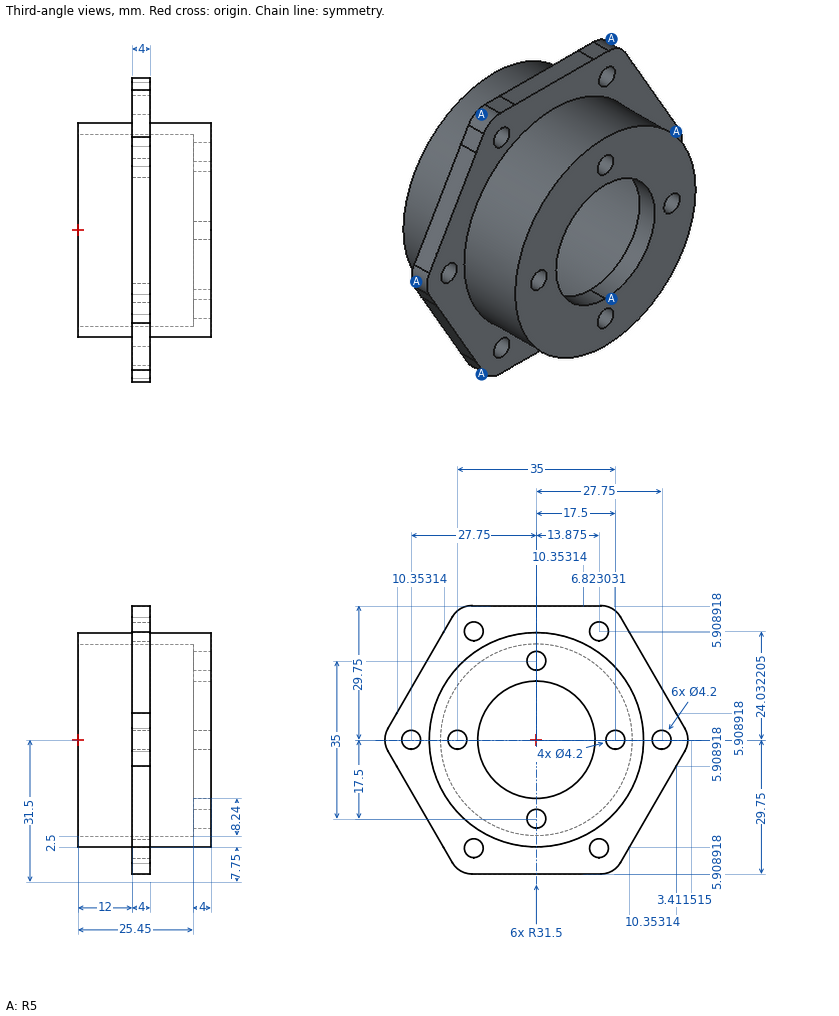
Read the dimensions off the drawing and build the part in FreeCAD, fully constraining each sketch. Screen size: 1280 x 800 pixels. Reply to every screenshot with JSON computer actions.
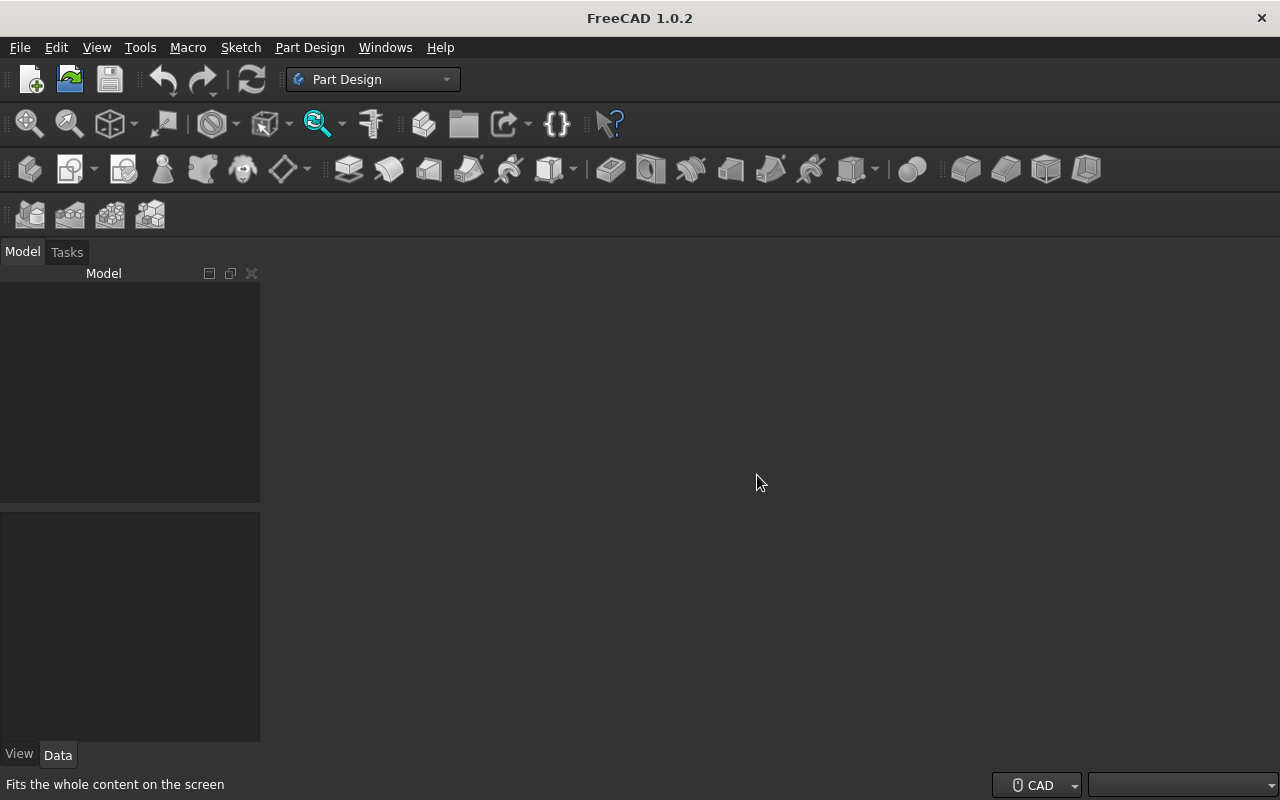
{"action": "key", "text": "ctrl+n"}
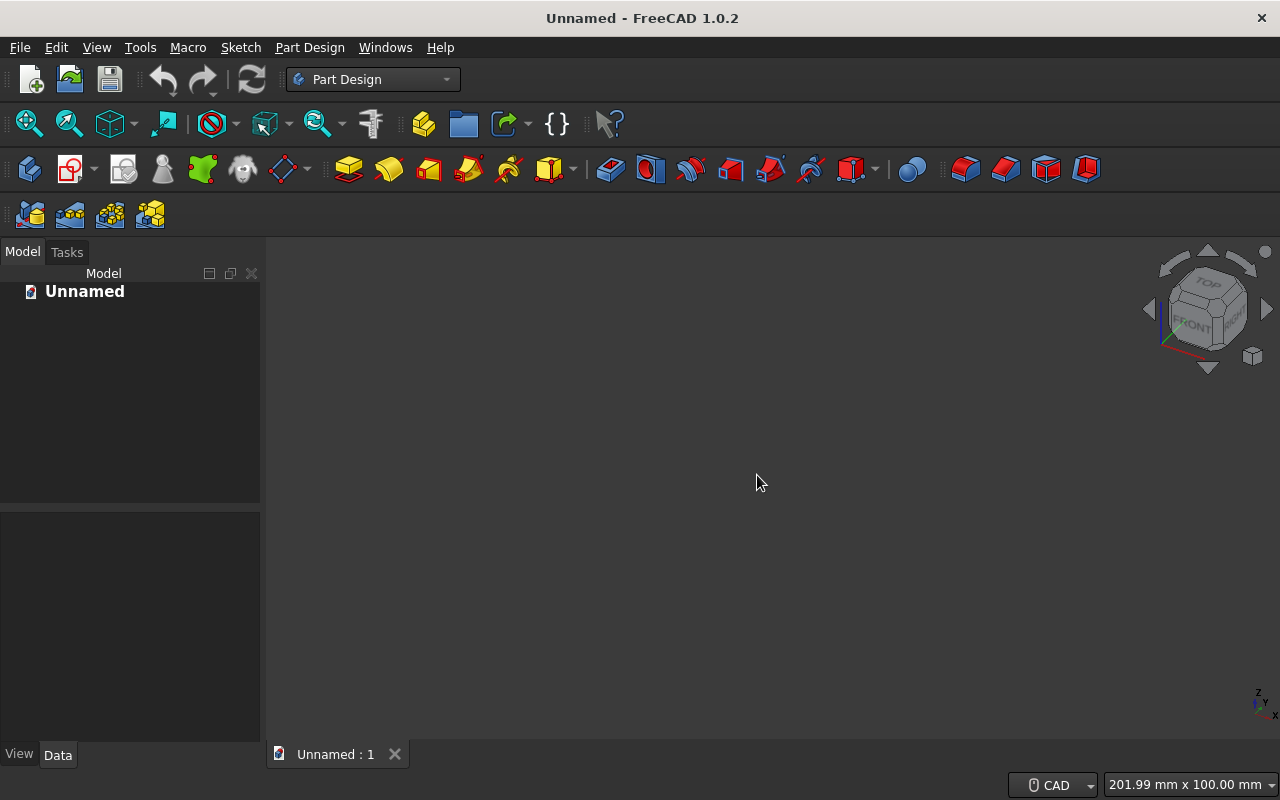
{"action": "left_click", "coordinate": [70, 170]}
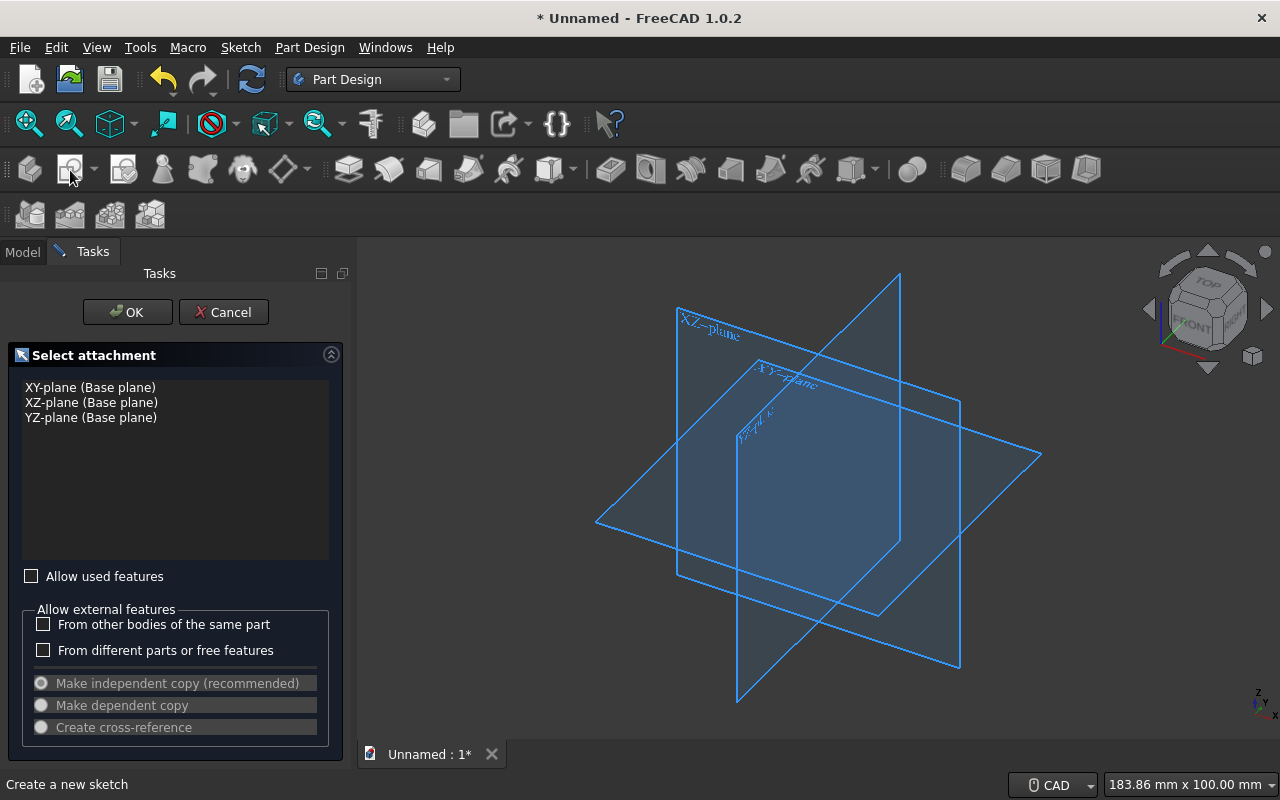
{"action": "left_click", "coordinate": [82, 402]}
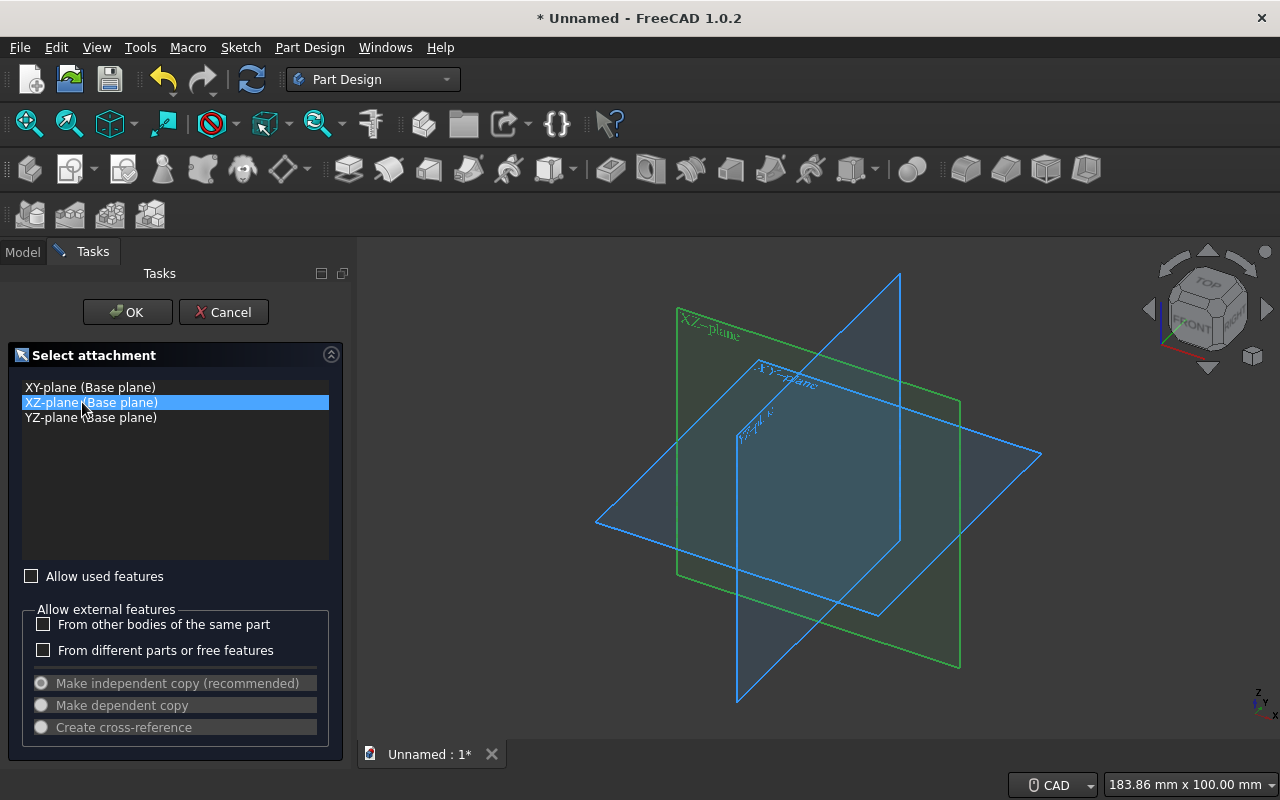
{"action": "left_click", "coordinate": [128, 312]}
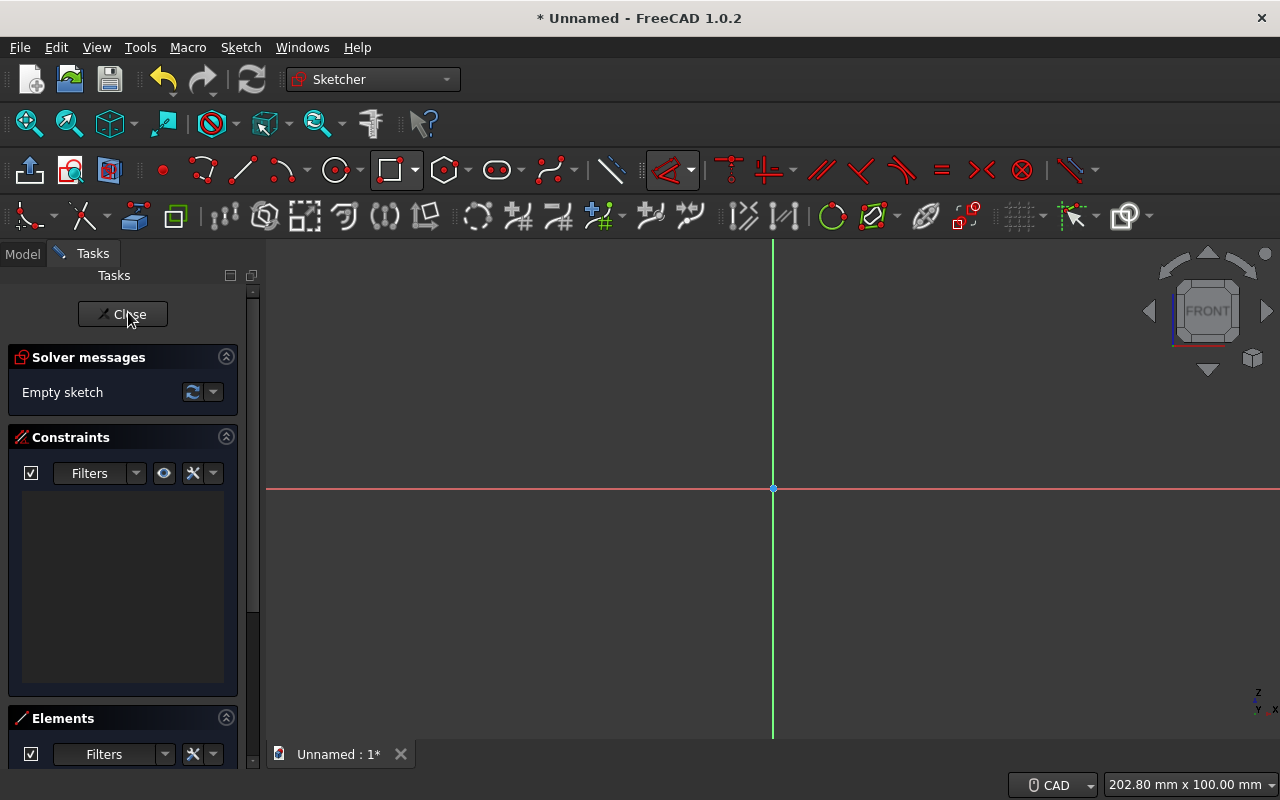
{"action": "scroll", "coordinate": [1020, 664], "scroll_direction": "up", "scroll_amount": 3}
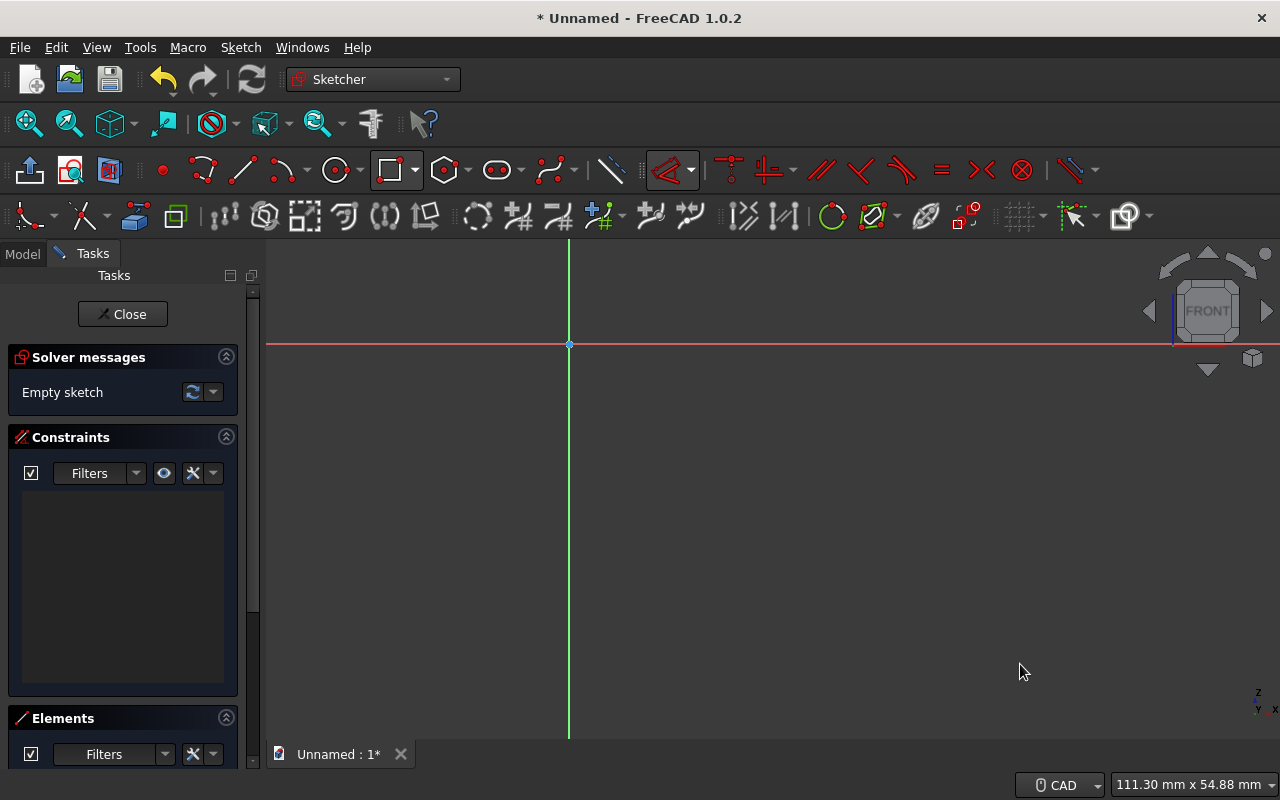
{"action": "key", "text": "g m"}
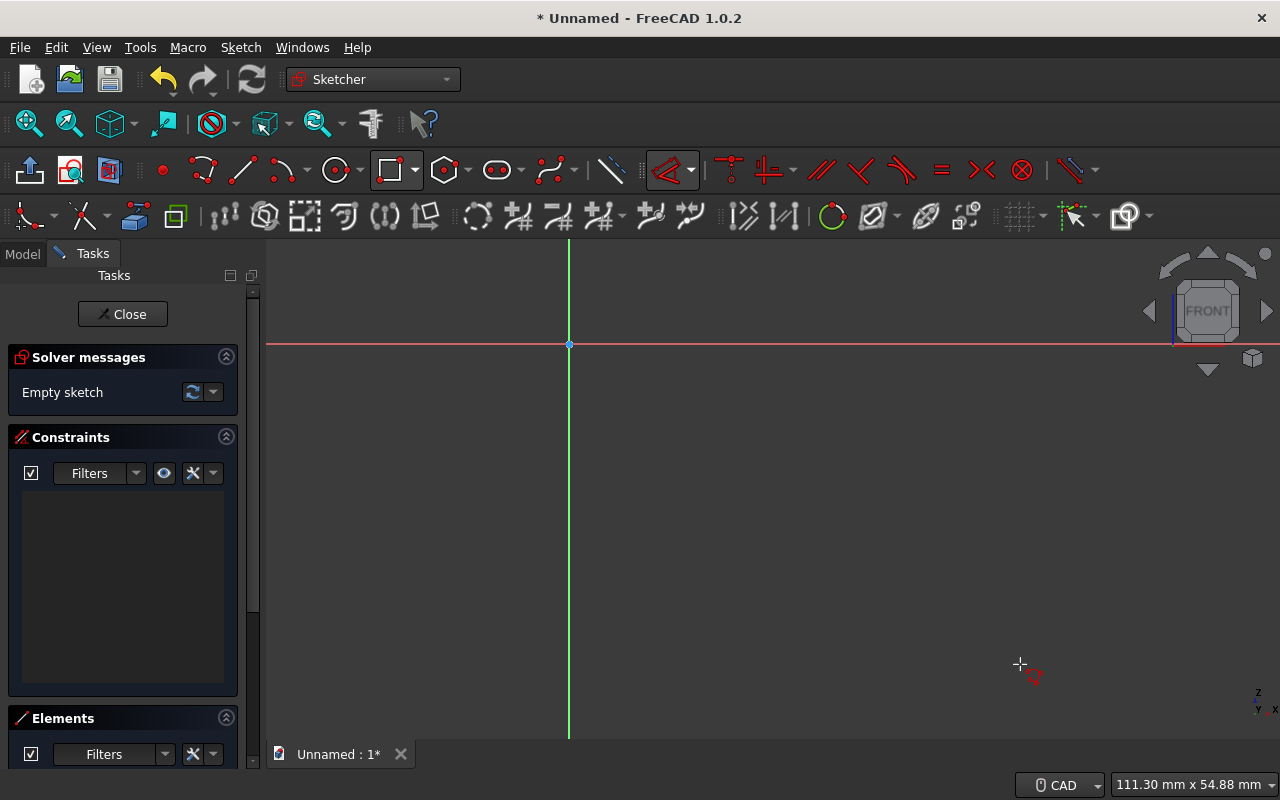
{"action": "left_click", "coordinate": [569, 538]}
{"action": "left_click", "coordinate": [801, 538]}
{"action": "left_click", "coordinate": [801, 463]}
{"action": "left_click", "coordinate": [838, 463]}
{"action": "left_click", "coordinate": [838, 561]}
{"action": "left_click", "coordinate": [715, 561]}
{"action": "left_click", "coordinate": [715, 631]}
{"action": "left_click", "coordinate": [679, 631]}
{"action": "left_click", "coordinate": [679, 561]}
{"action": "left_click", "coordinate": [578, 561]}
{"action": "left_click", "coordinate": [569, 539]}
{"action": "key", "text": "Escape"}
{"action": "key", "text": "Escape"}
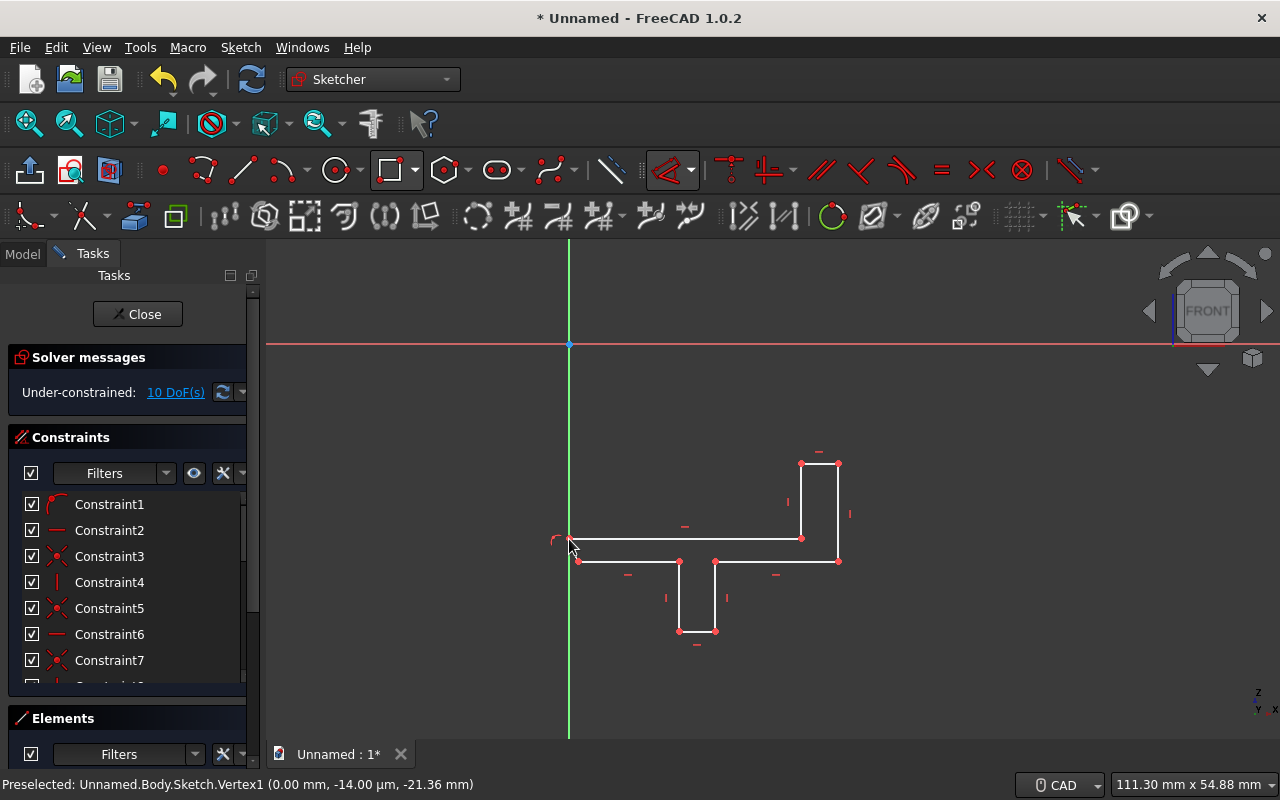
{"action": "scroll", "coordinate": [573, 548], "scroll_direction": "up", "scroll_amount": 3}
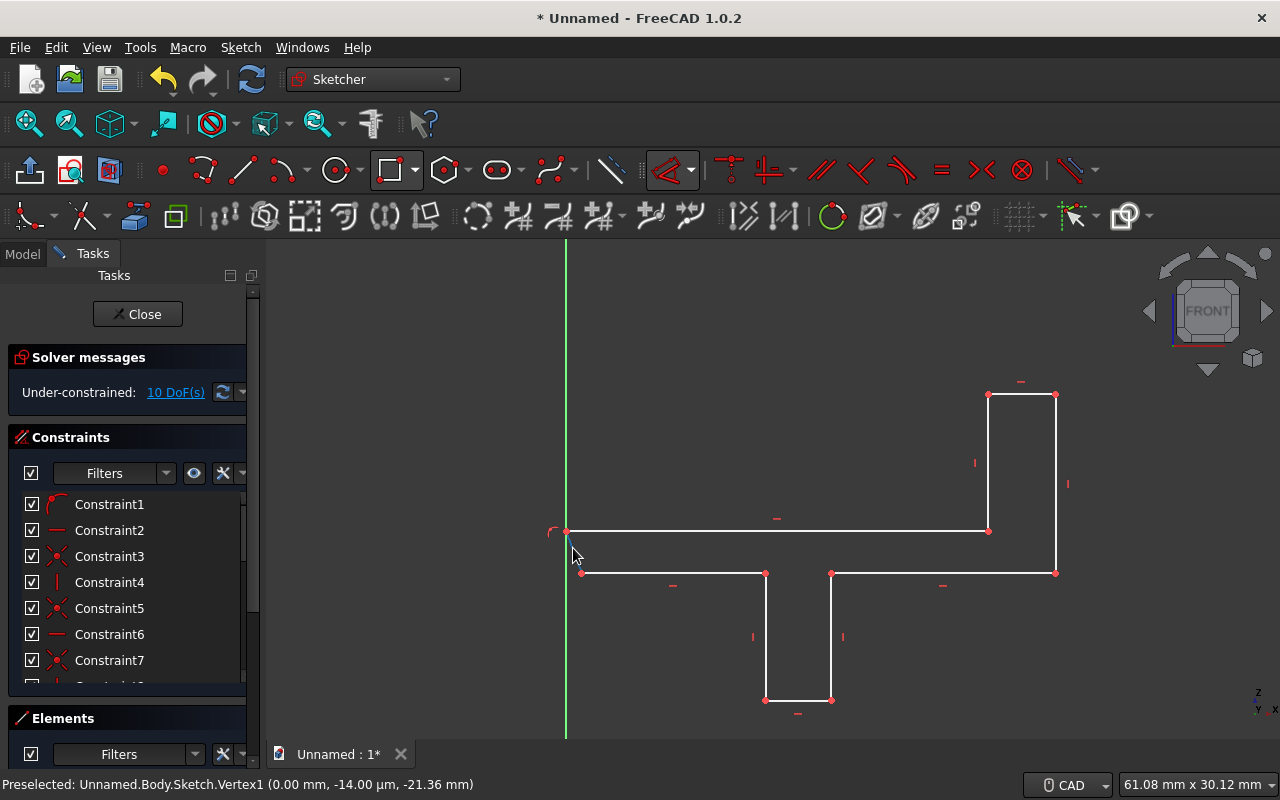
{"action": "left_click", "coordinate": [572, 548]}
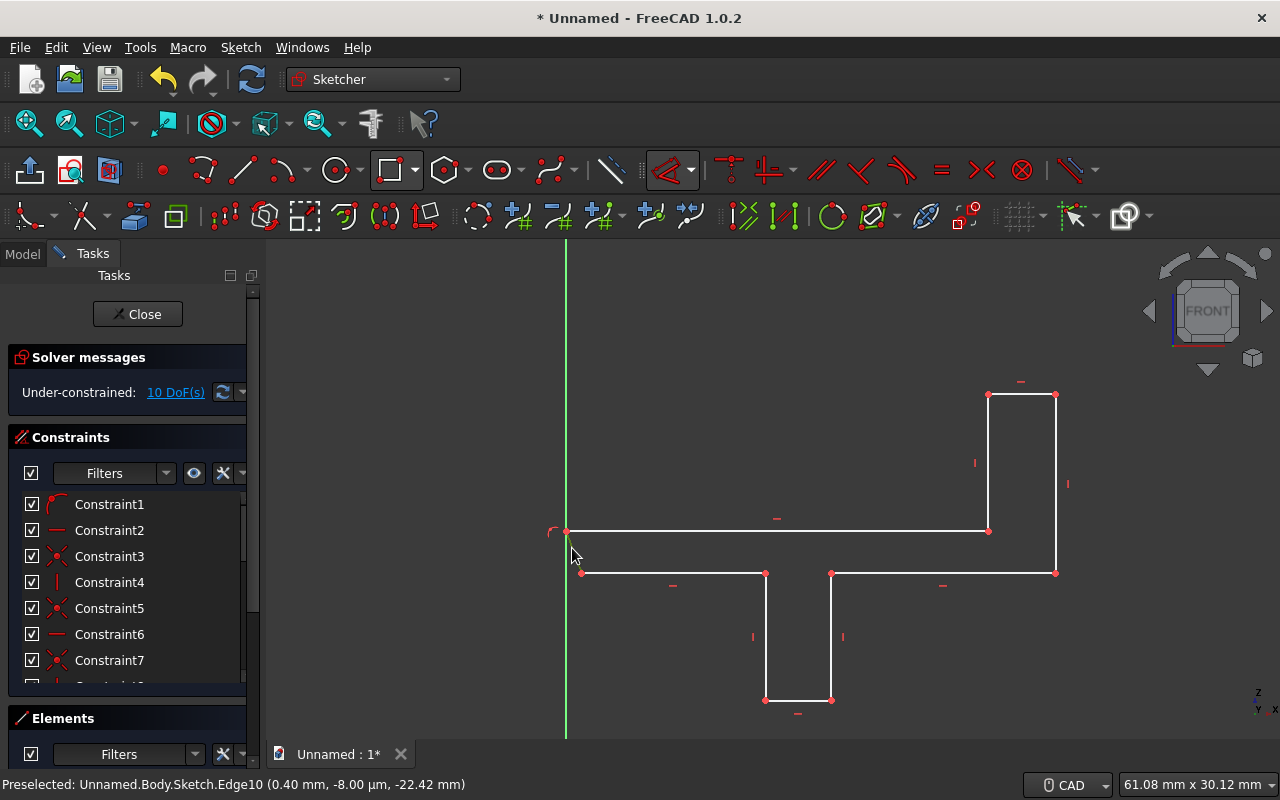
{"action": "key", "text": "v"}